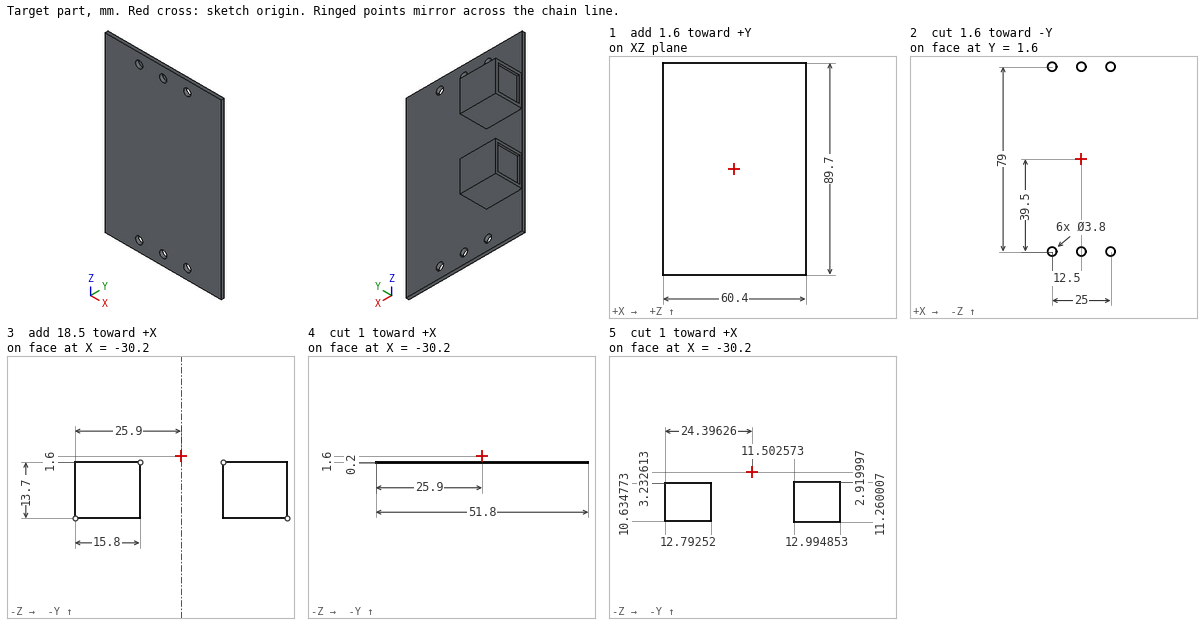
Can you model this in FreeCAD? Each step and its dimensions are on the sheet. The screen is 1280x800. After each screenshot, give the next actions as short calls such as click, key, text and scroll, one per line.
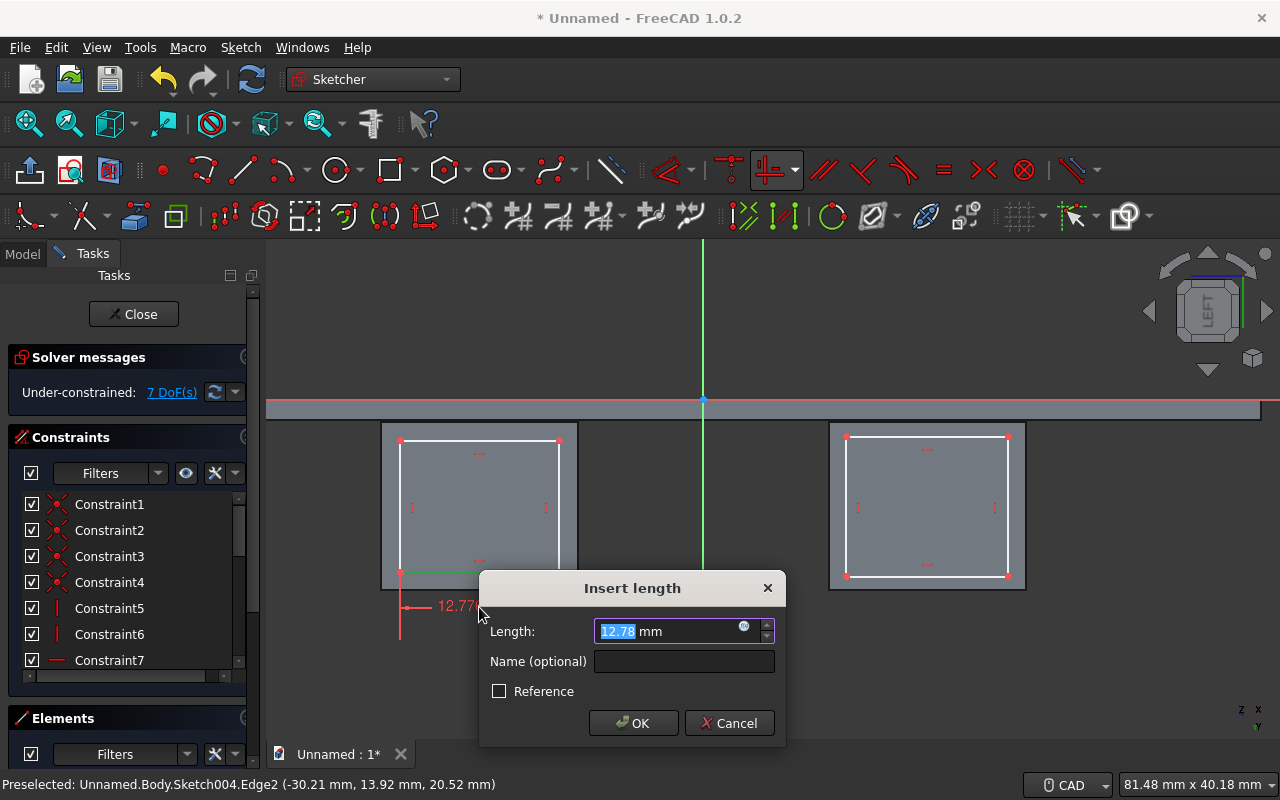
text(12.79252)
key(Return)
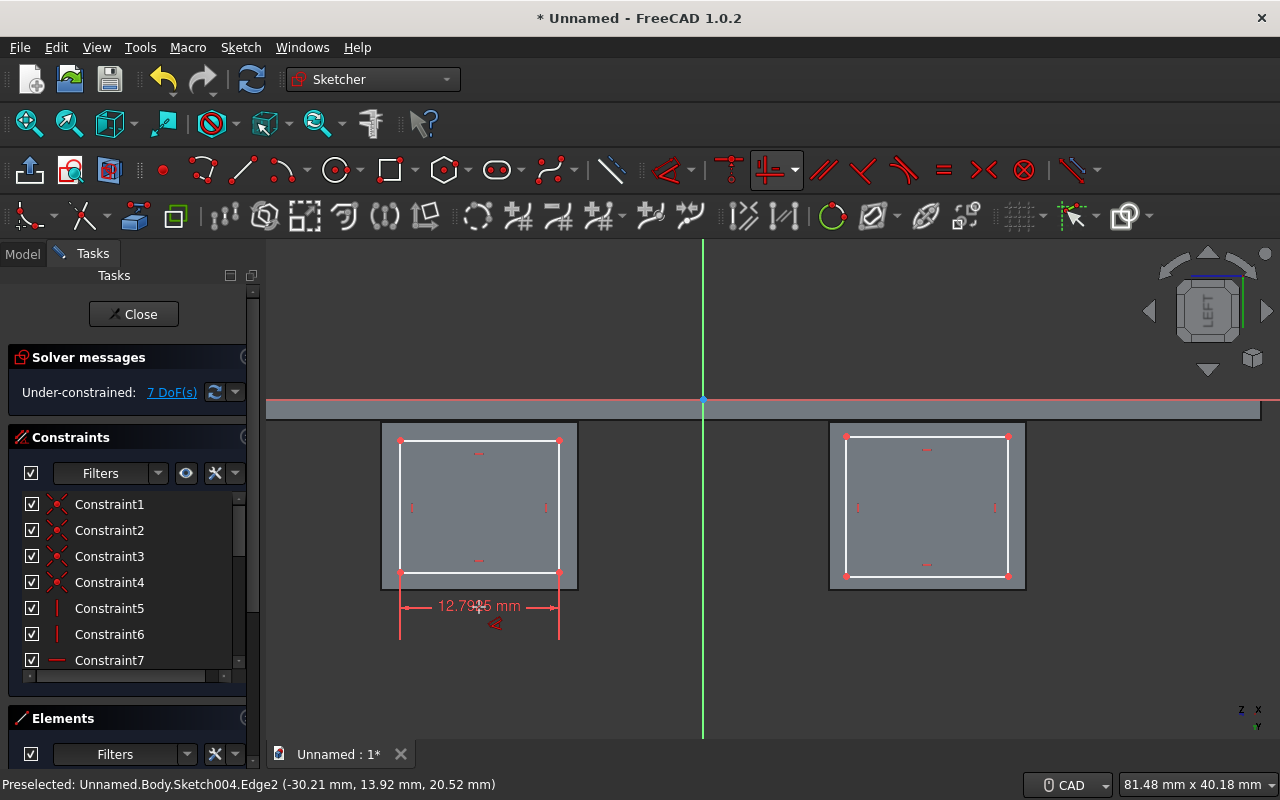
click(400, 481)
click(366, 507)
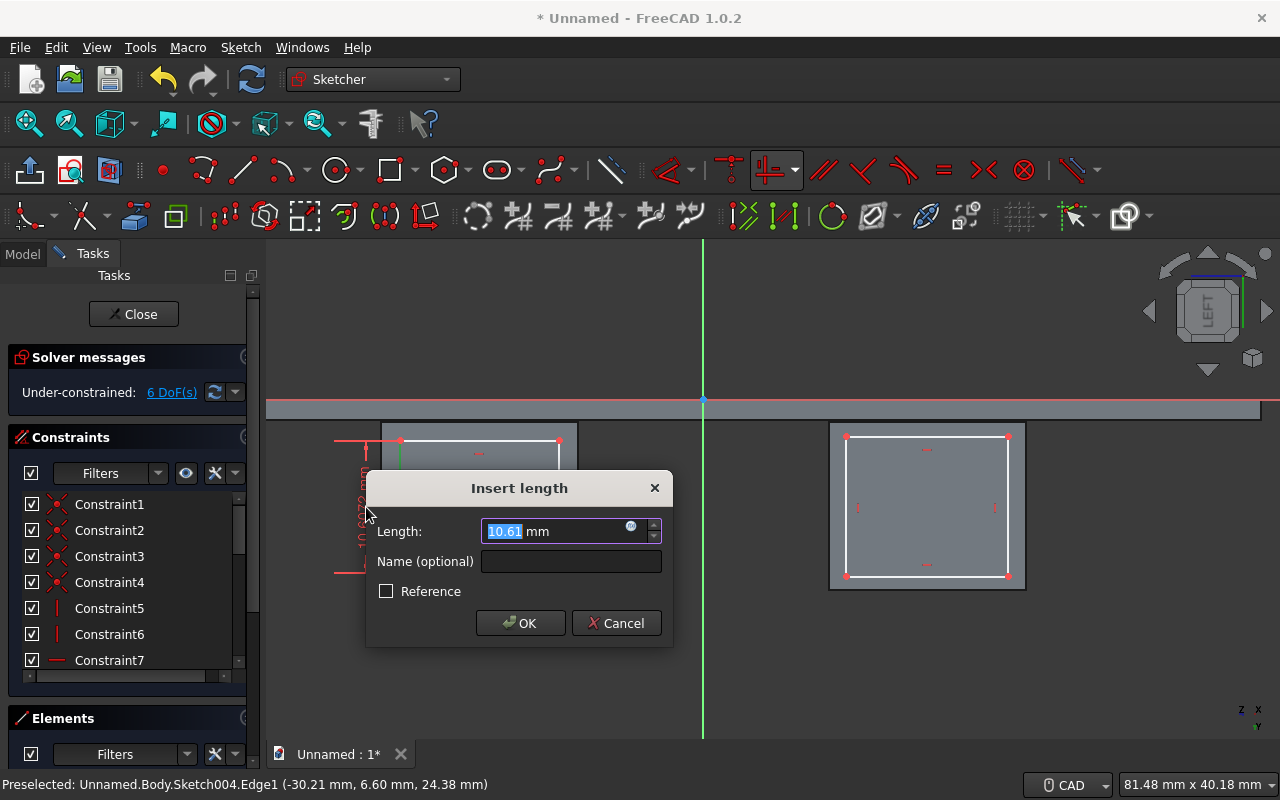
text(10.634773)
key(Return)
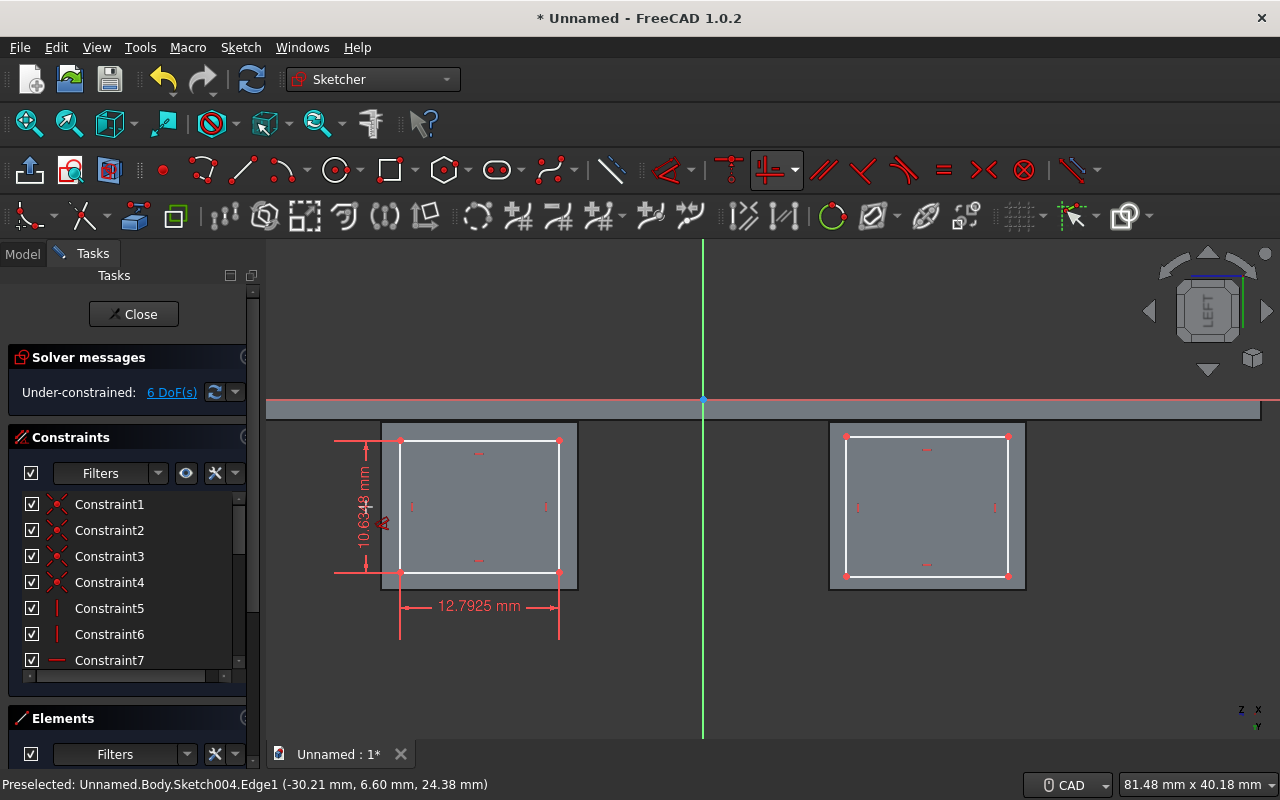
click(846, 479)
click(880, 507)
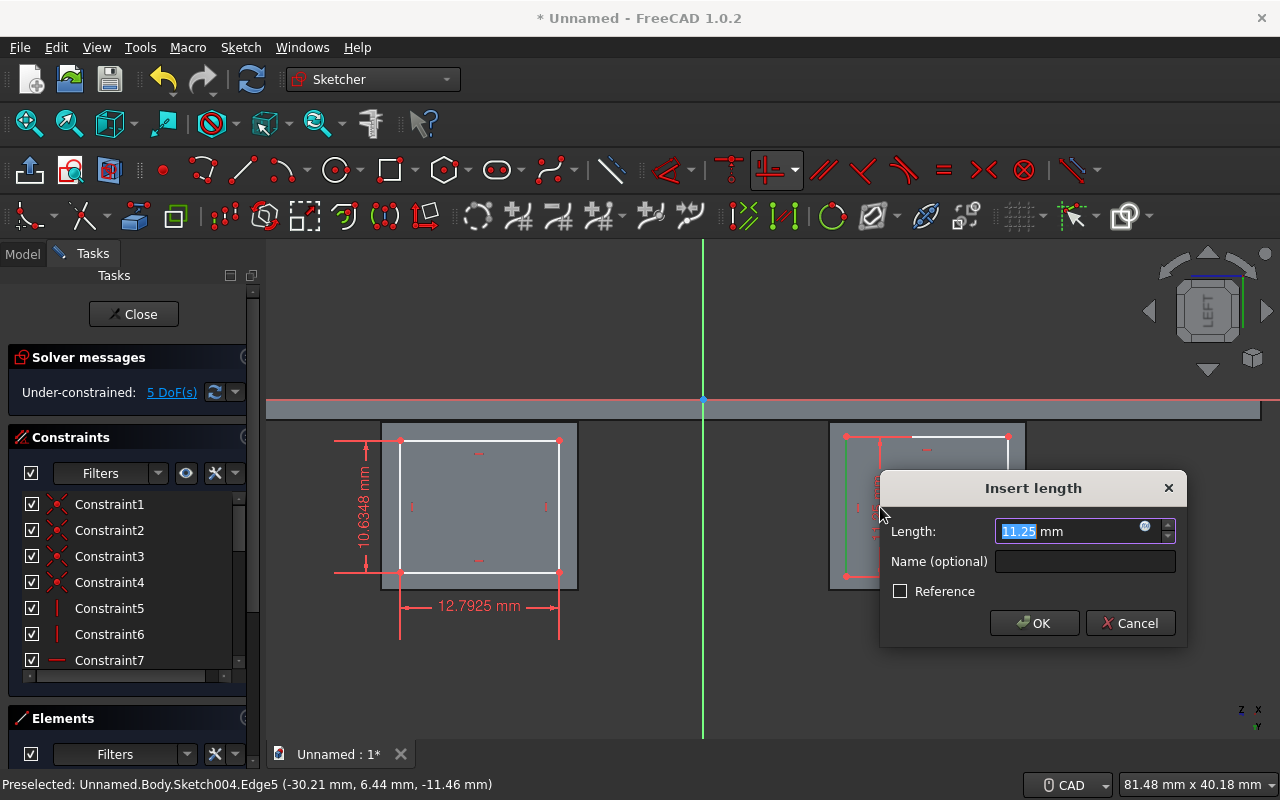
text(11.260007)
key(Return)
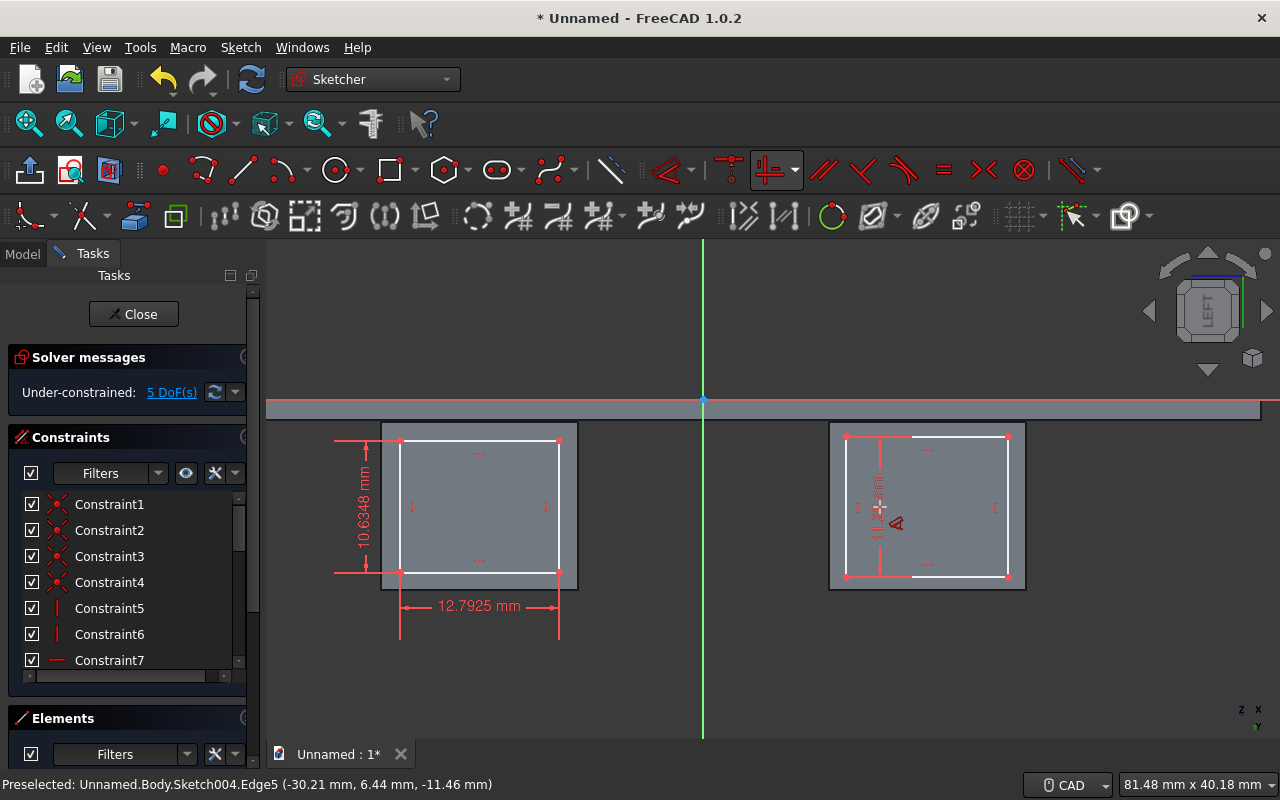
click(895, 577)
click(927, 611)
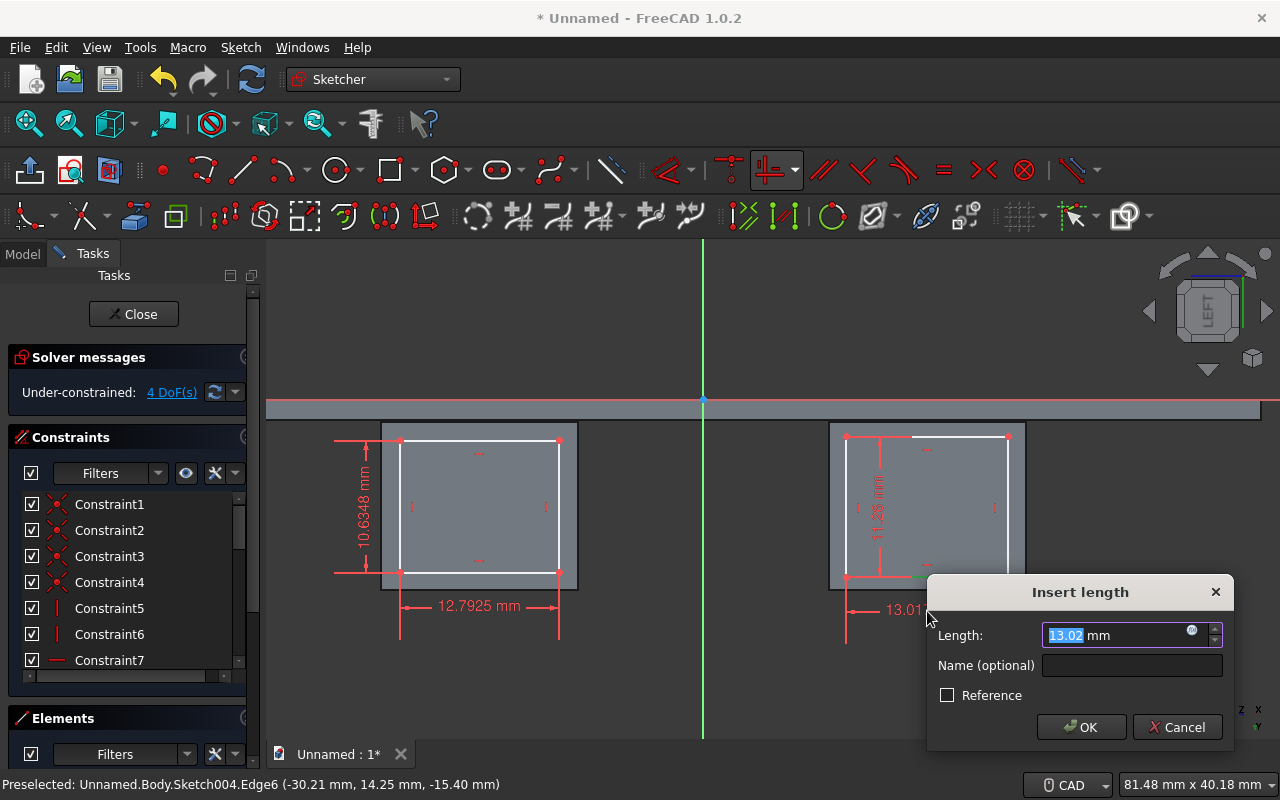
text(12.994853)
key(Return)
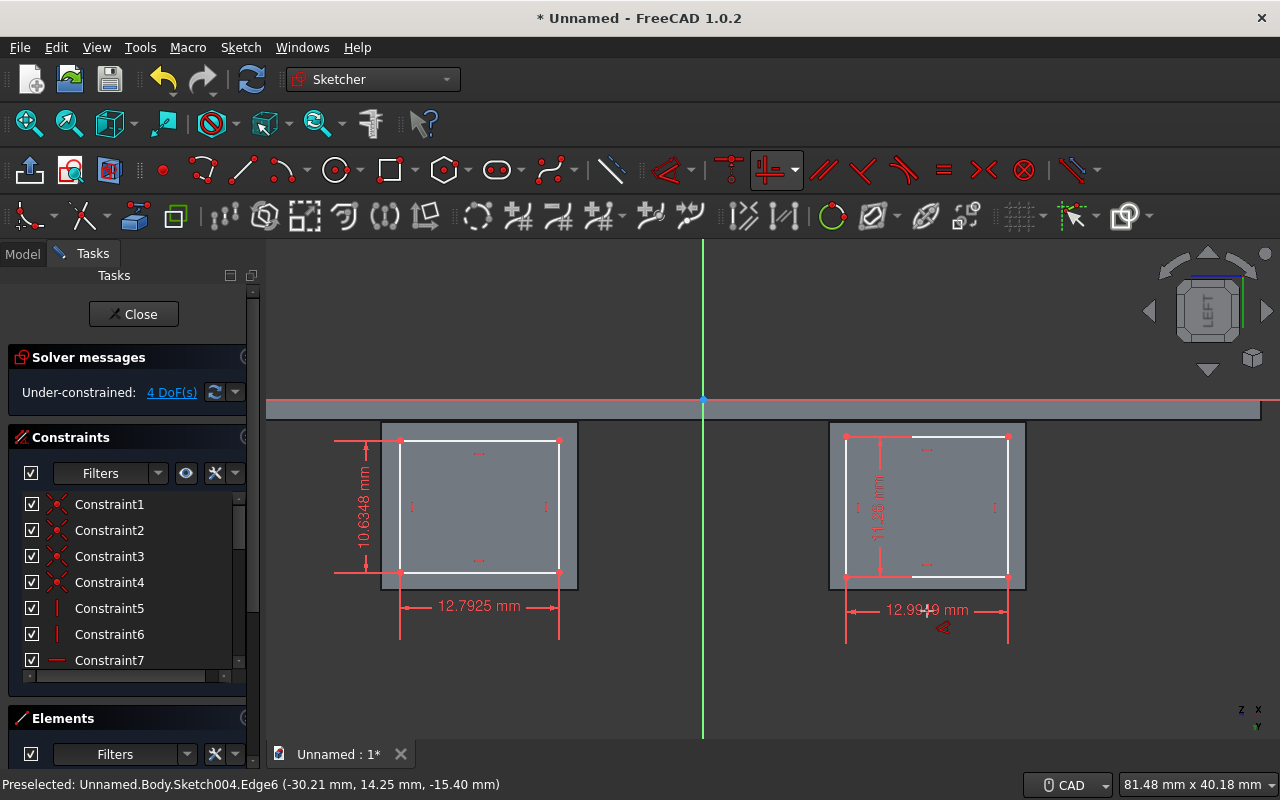
click(400, 441)
click(552, 366)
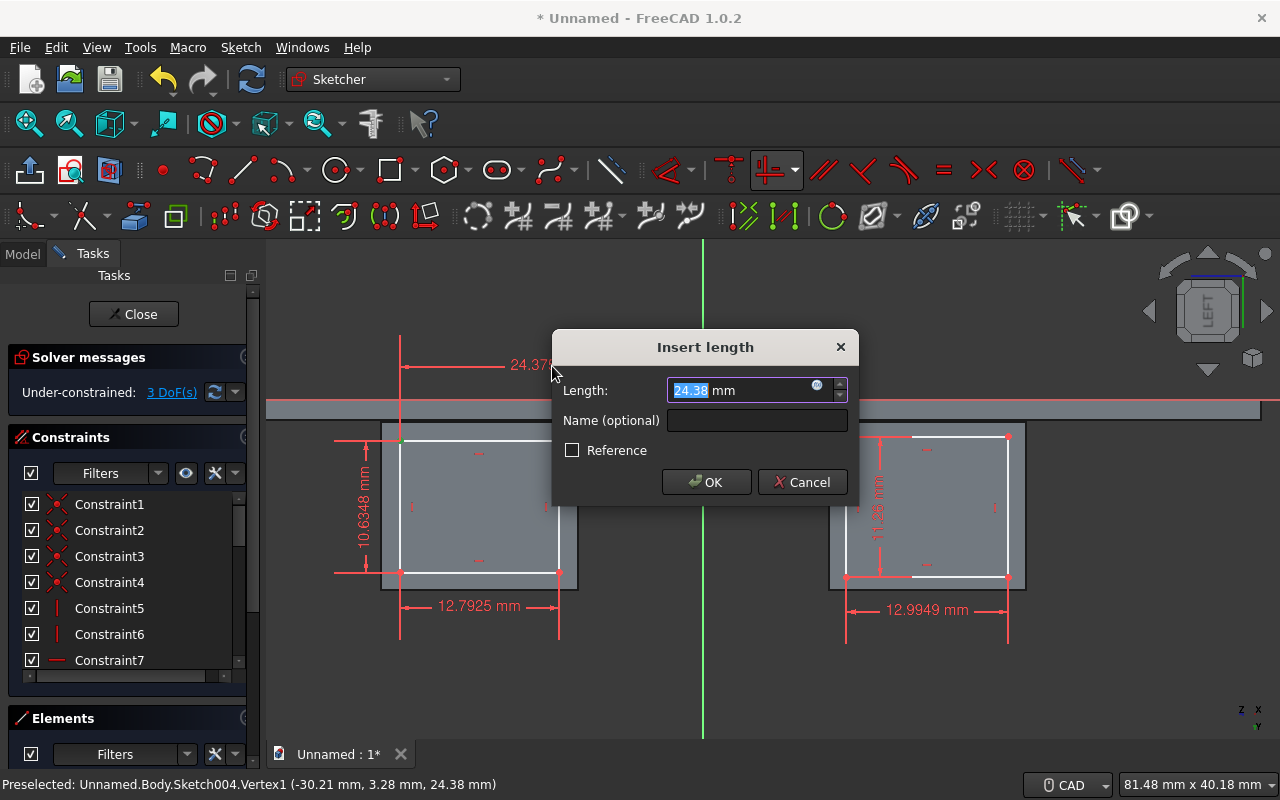
text(24.39626)
key(Return)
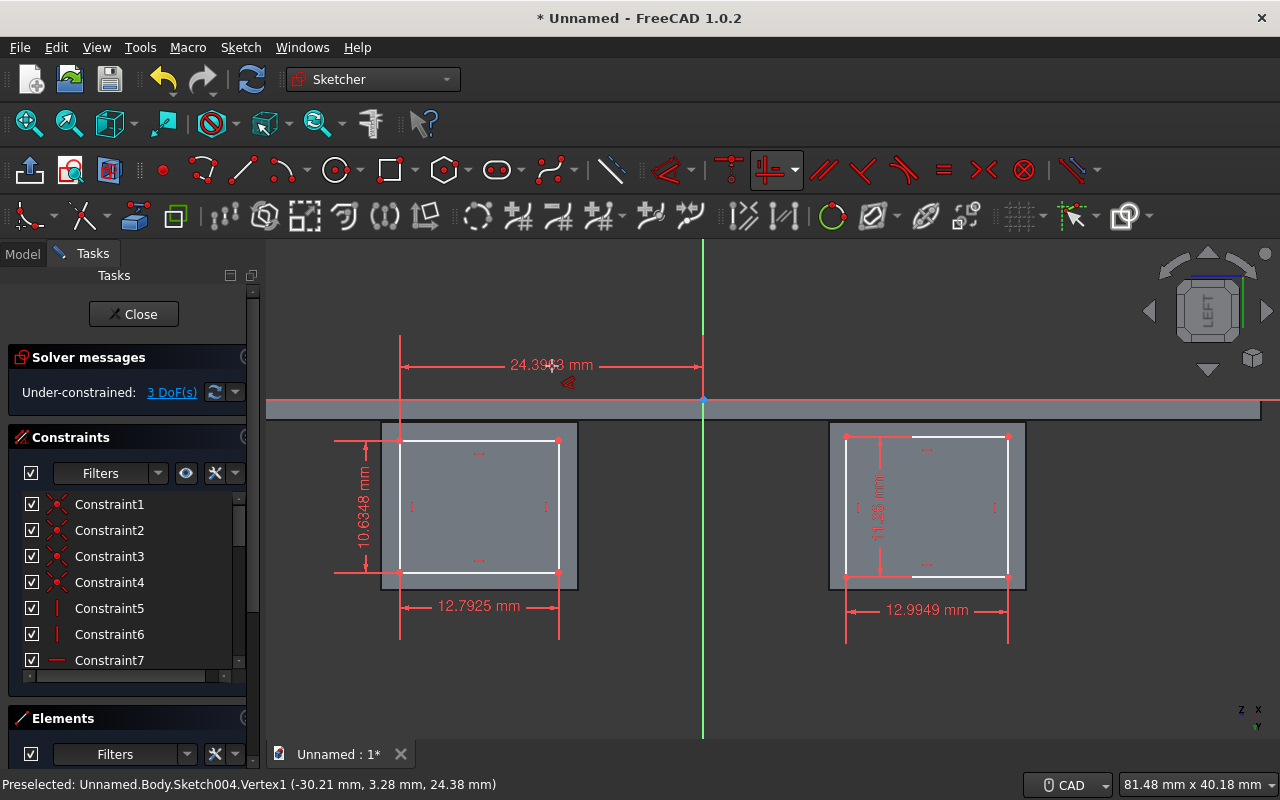
click(400, 441)
click(366, 420)